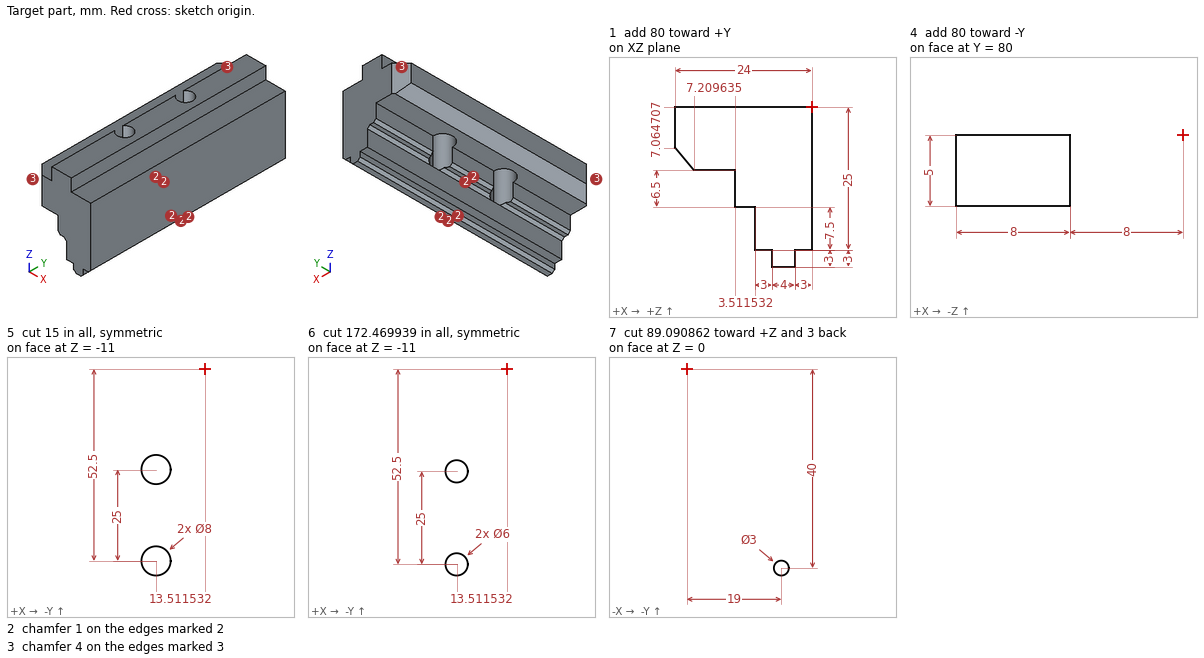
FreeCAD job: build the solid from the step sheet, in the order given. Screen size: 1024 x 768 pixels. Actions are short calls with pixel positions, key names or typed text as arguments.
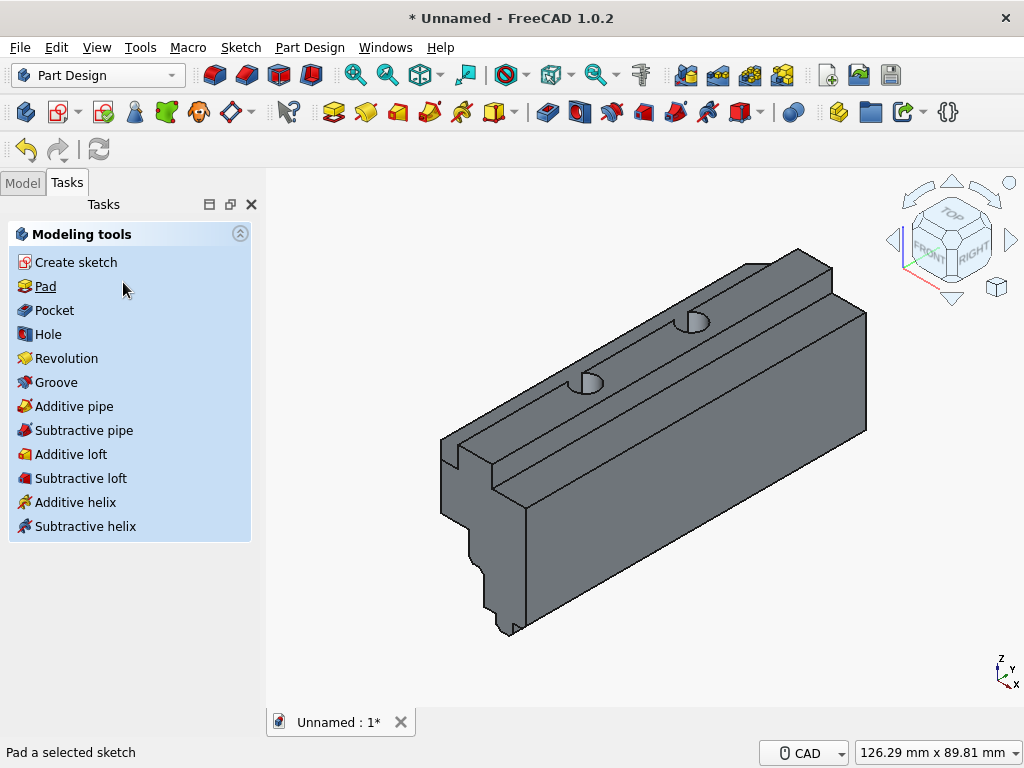
click(548, 112)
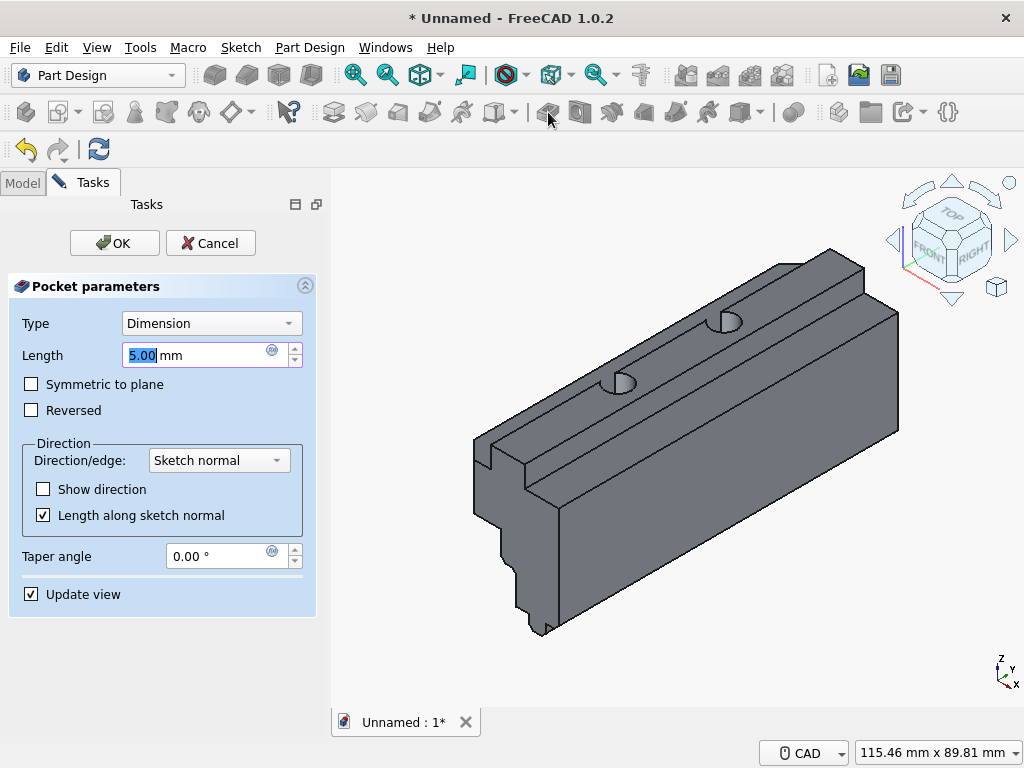
click(212, 324)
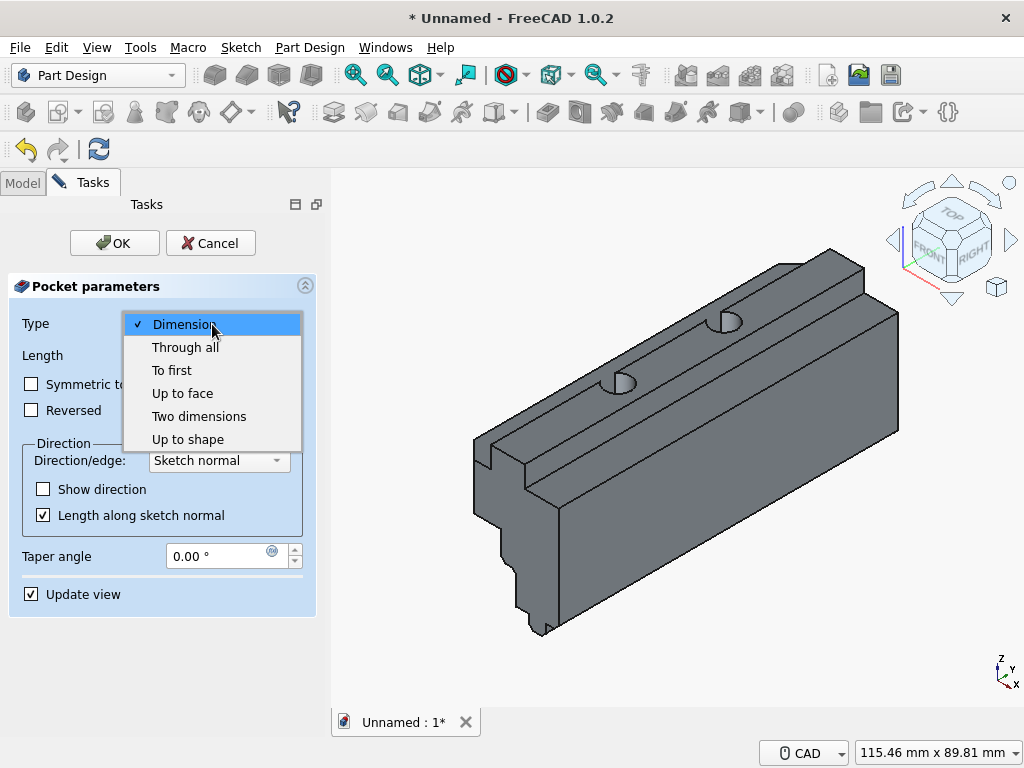
click(212, 416)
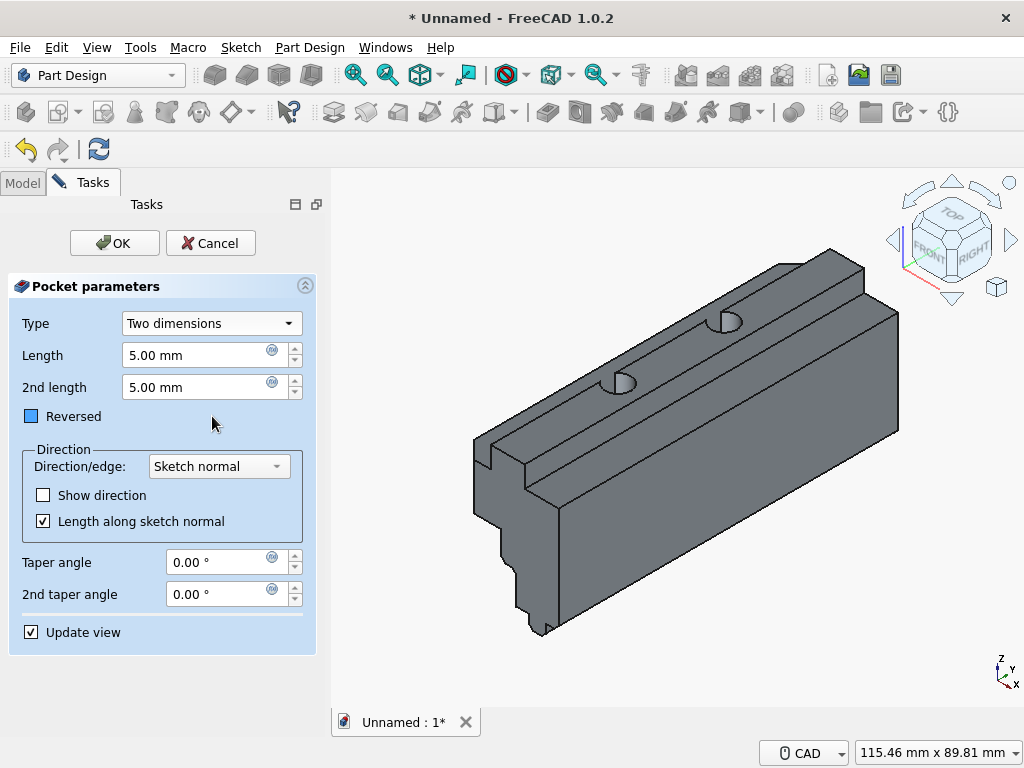
triple_click(204, 355)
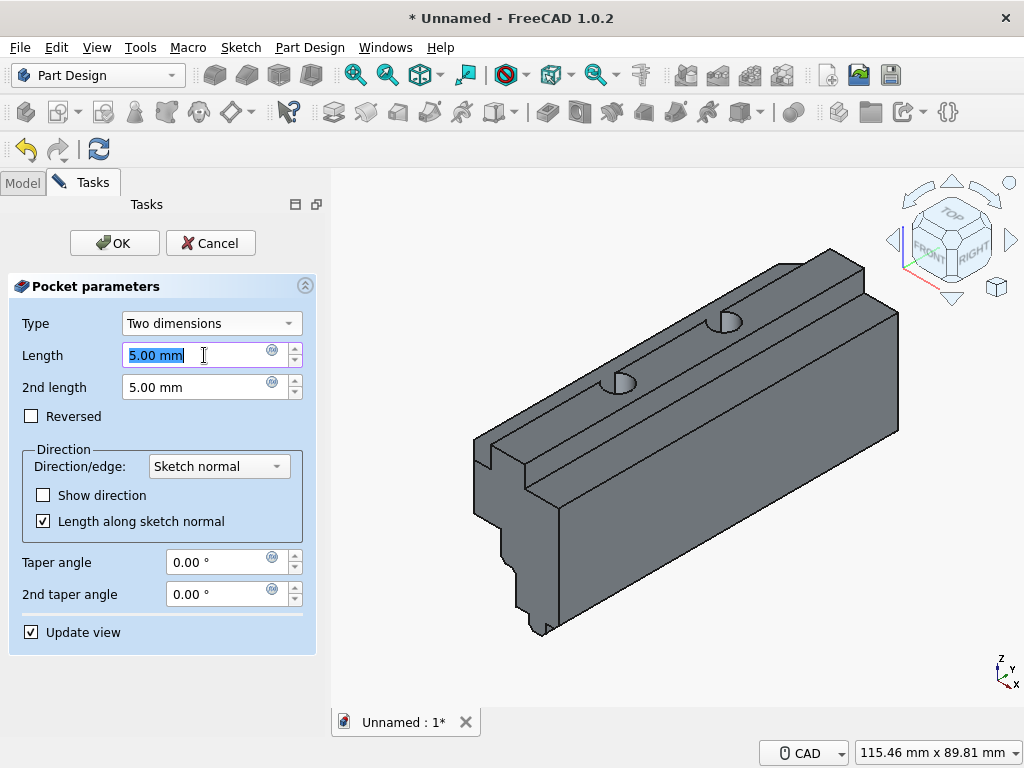
text(89.090862)
key(Tab)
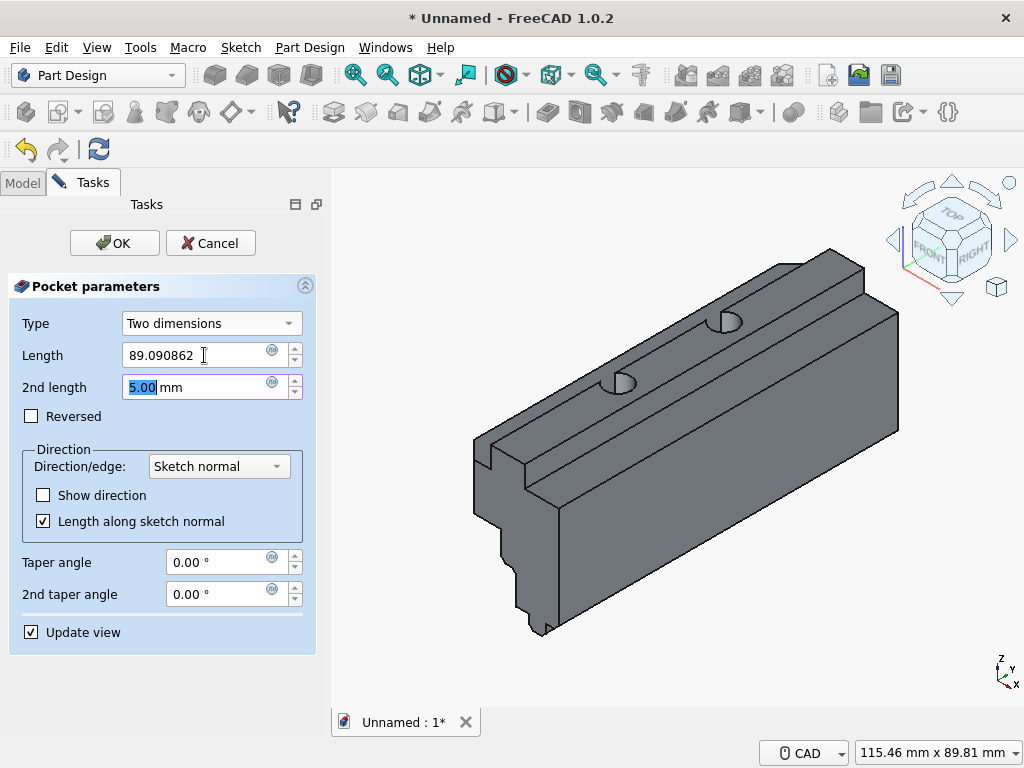
text(3)
key(Tab)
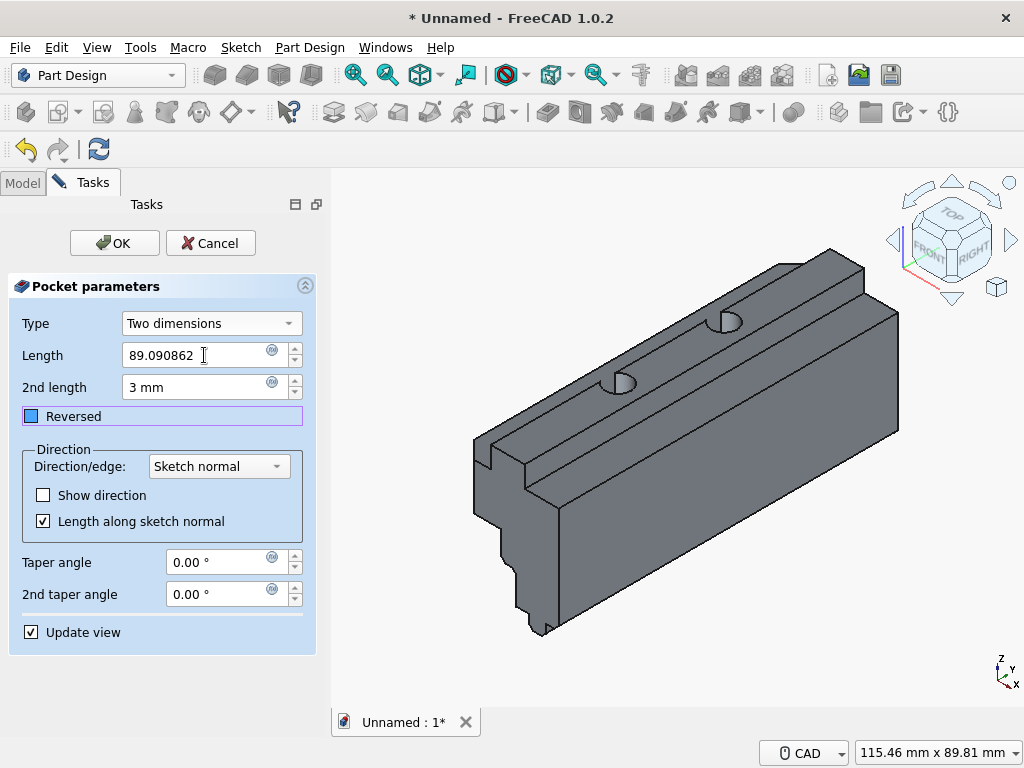
click(30, 416)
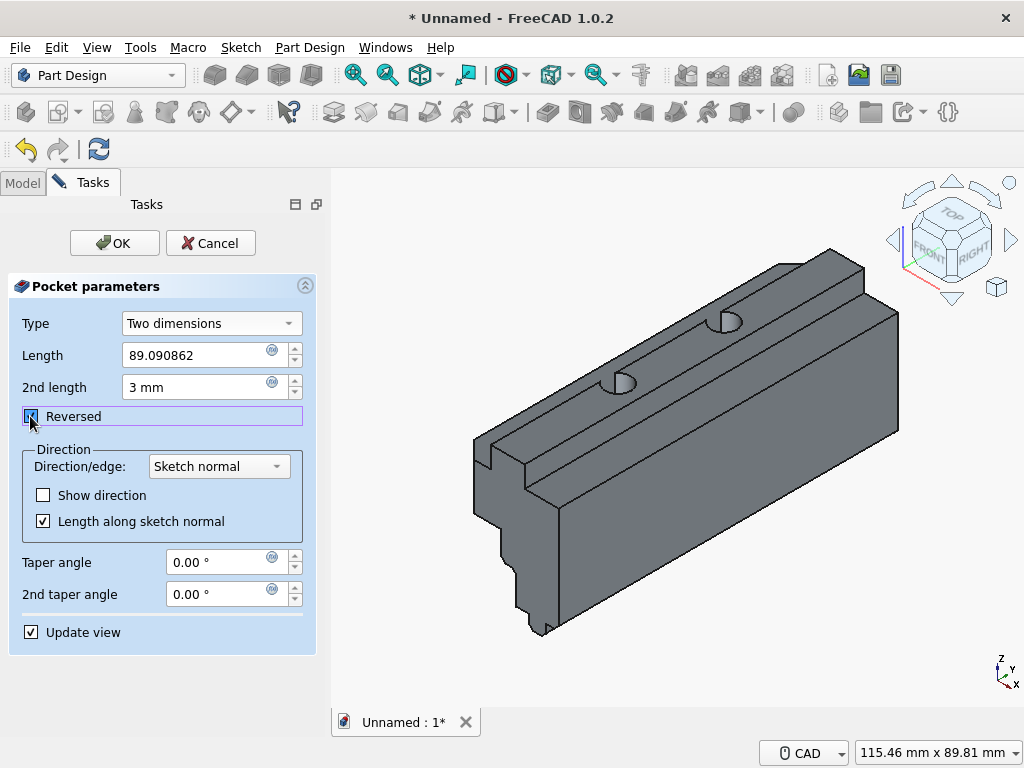
click(115, 243)